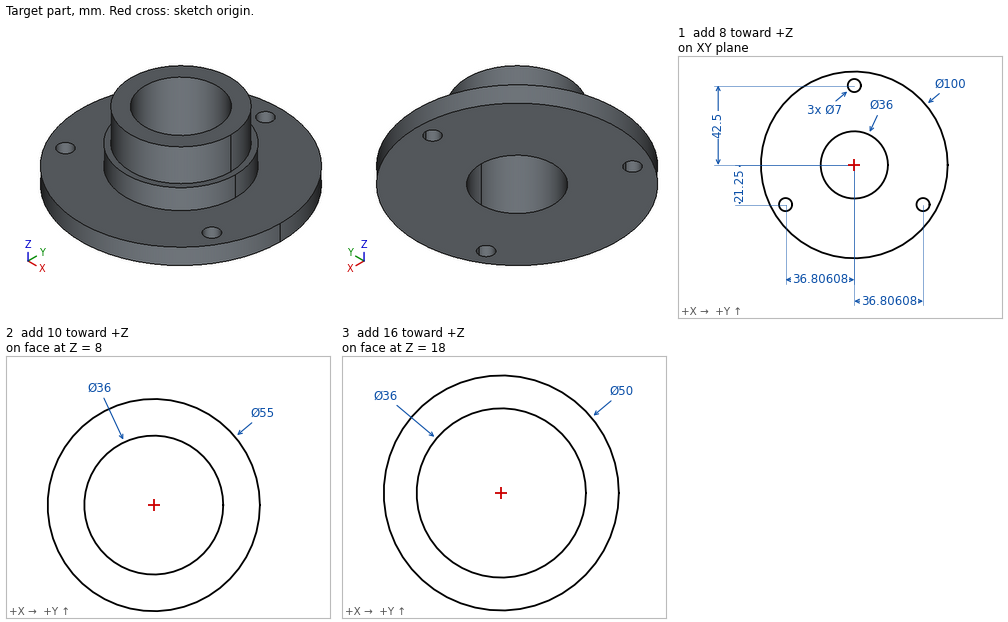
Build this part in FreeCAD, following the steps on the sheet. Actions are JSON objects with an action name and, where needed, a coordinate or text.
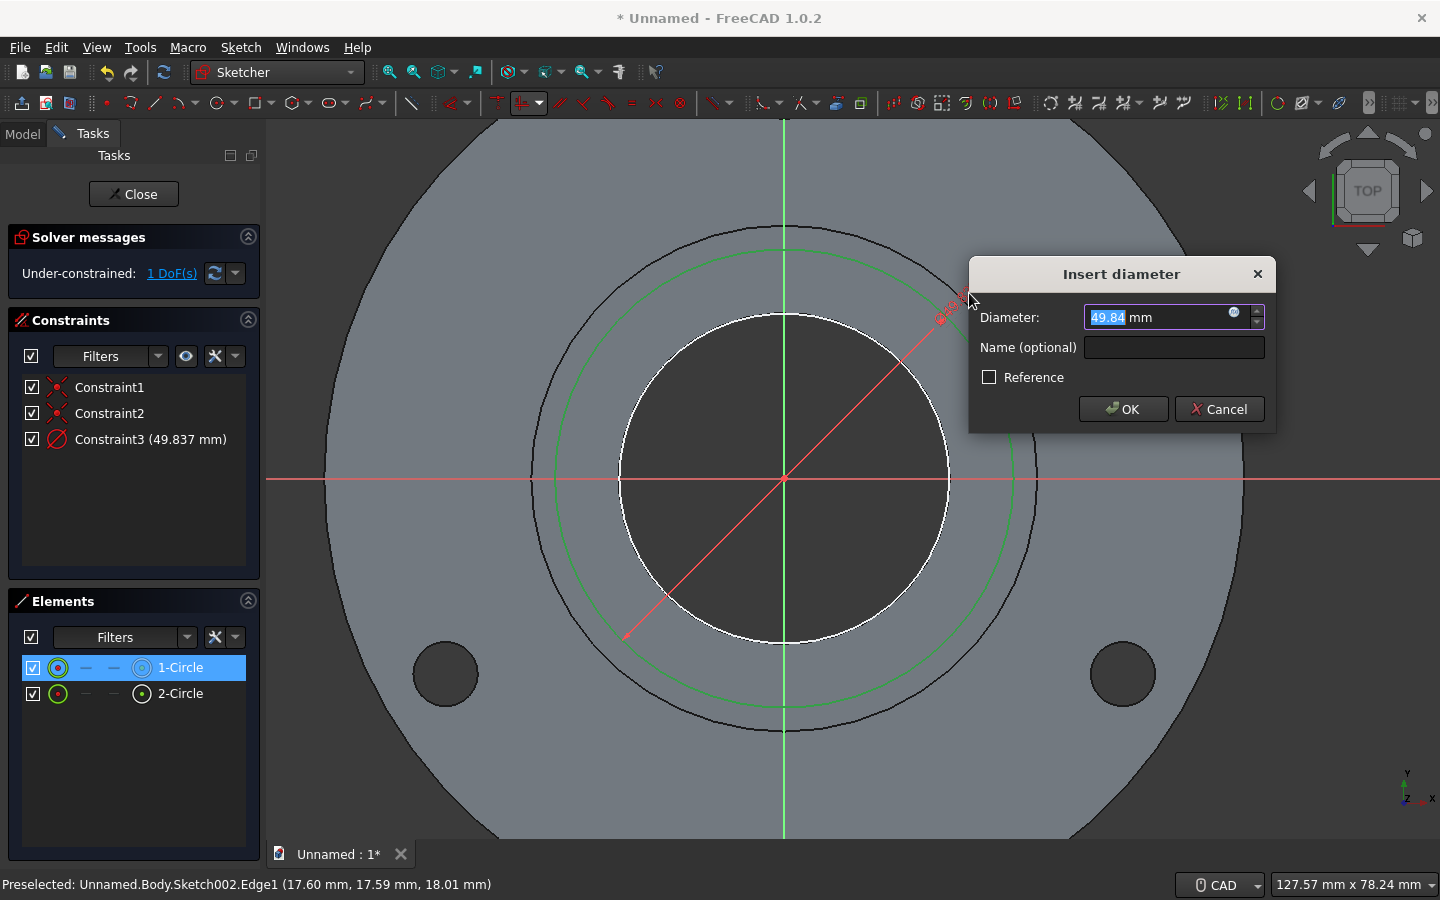
{"action": "type", "text": "50"}
{"action": "key", "text": "Return"}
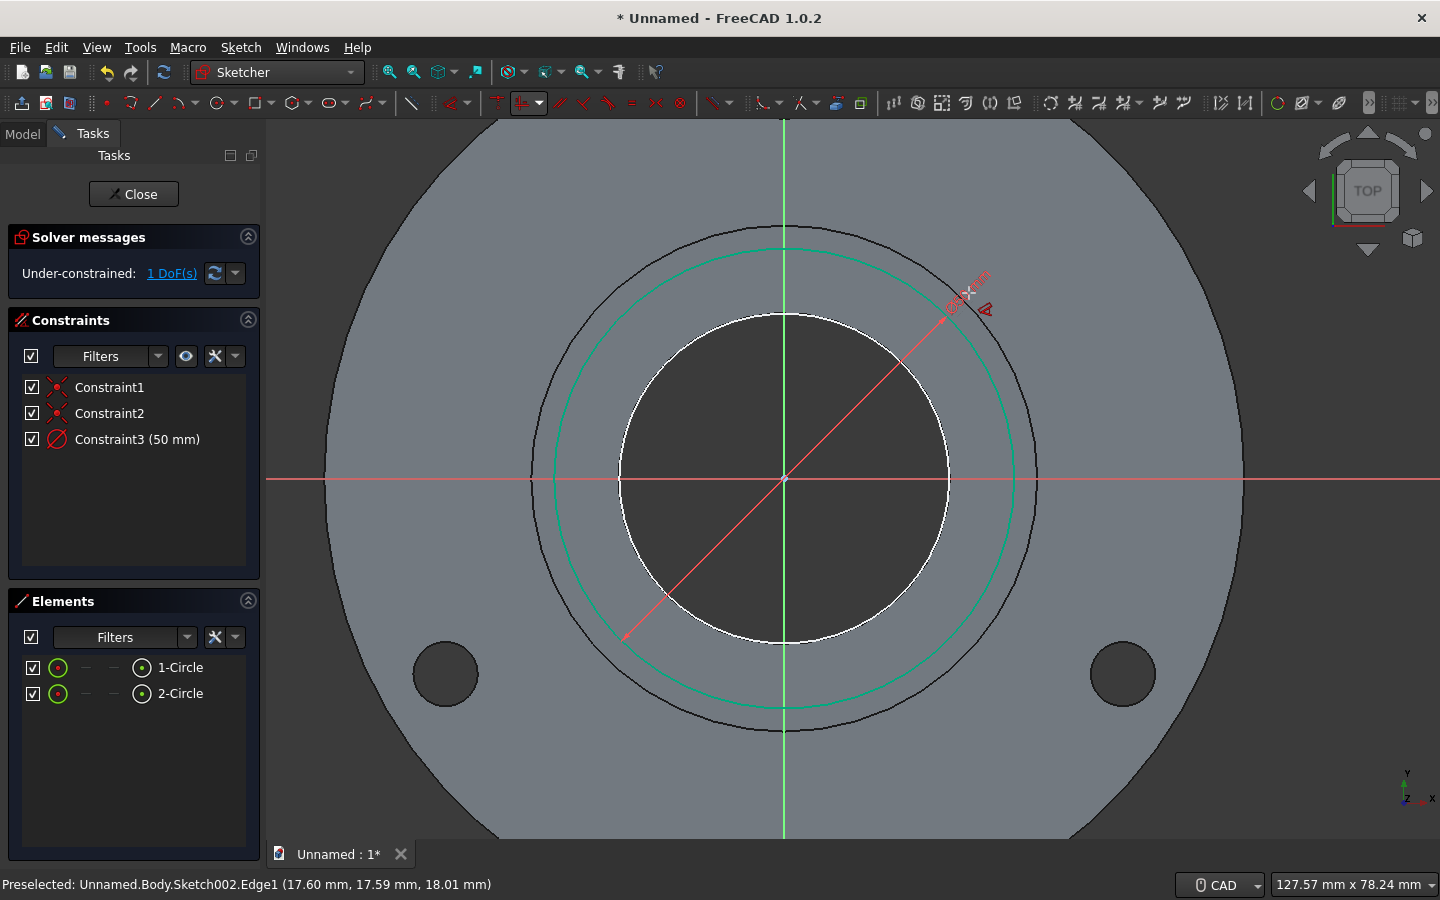
{"action": "left_click", "coordinate": [901, 362]}
{"action": "left_click", "coordinate": [924, 339]}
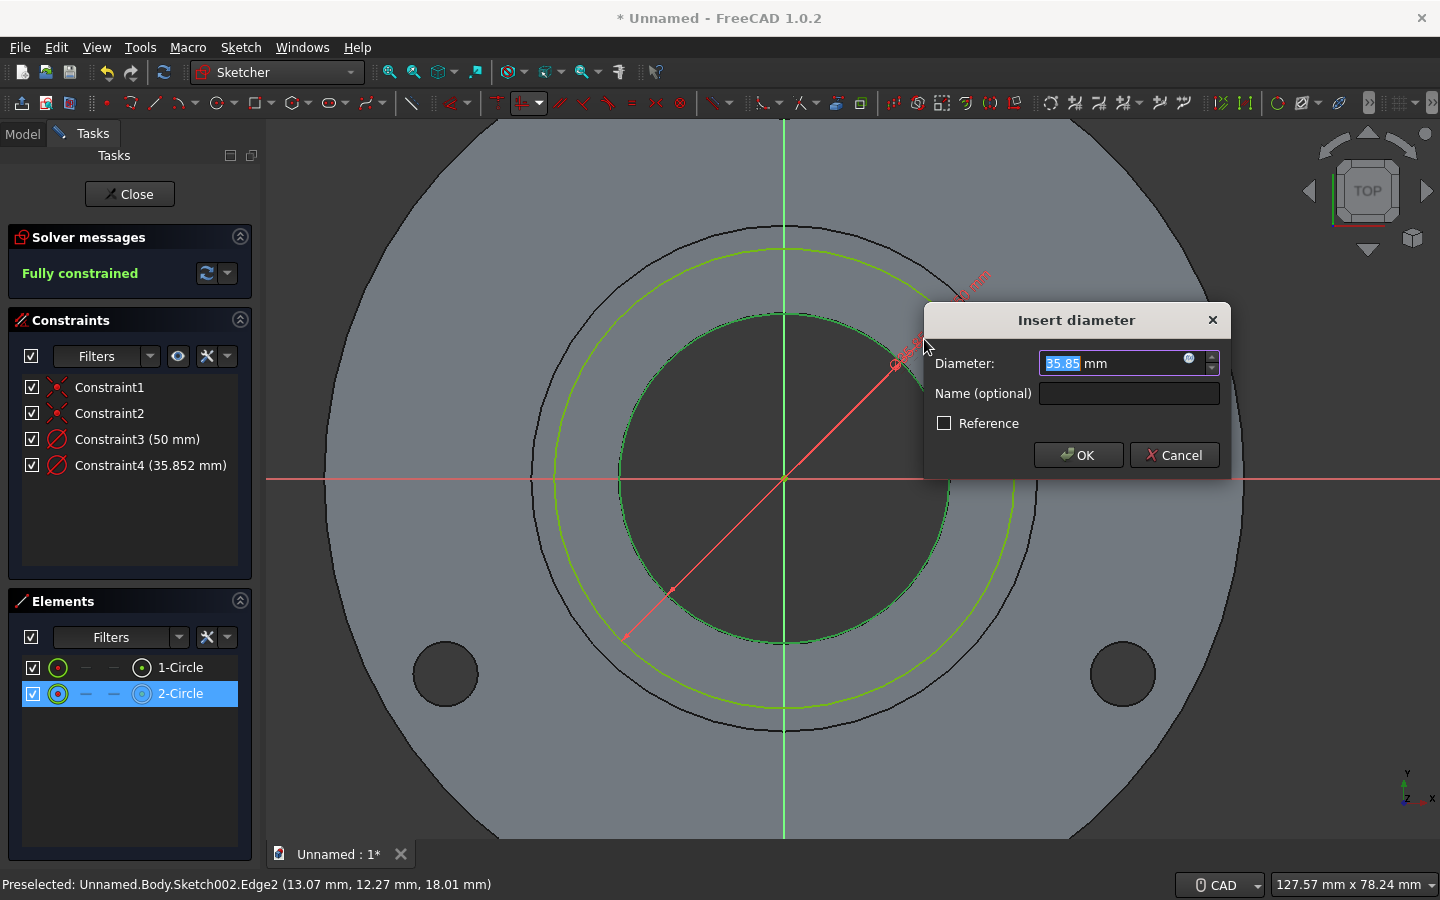
{"action": "type", "text": "36"}
{"action": "key", "text": "Return"}
{"action": "key", "text": "Escape"}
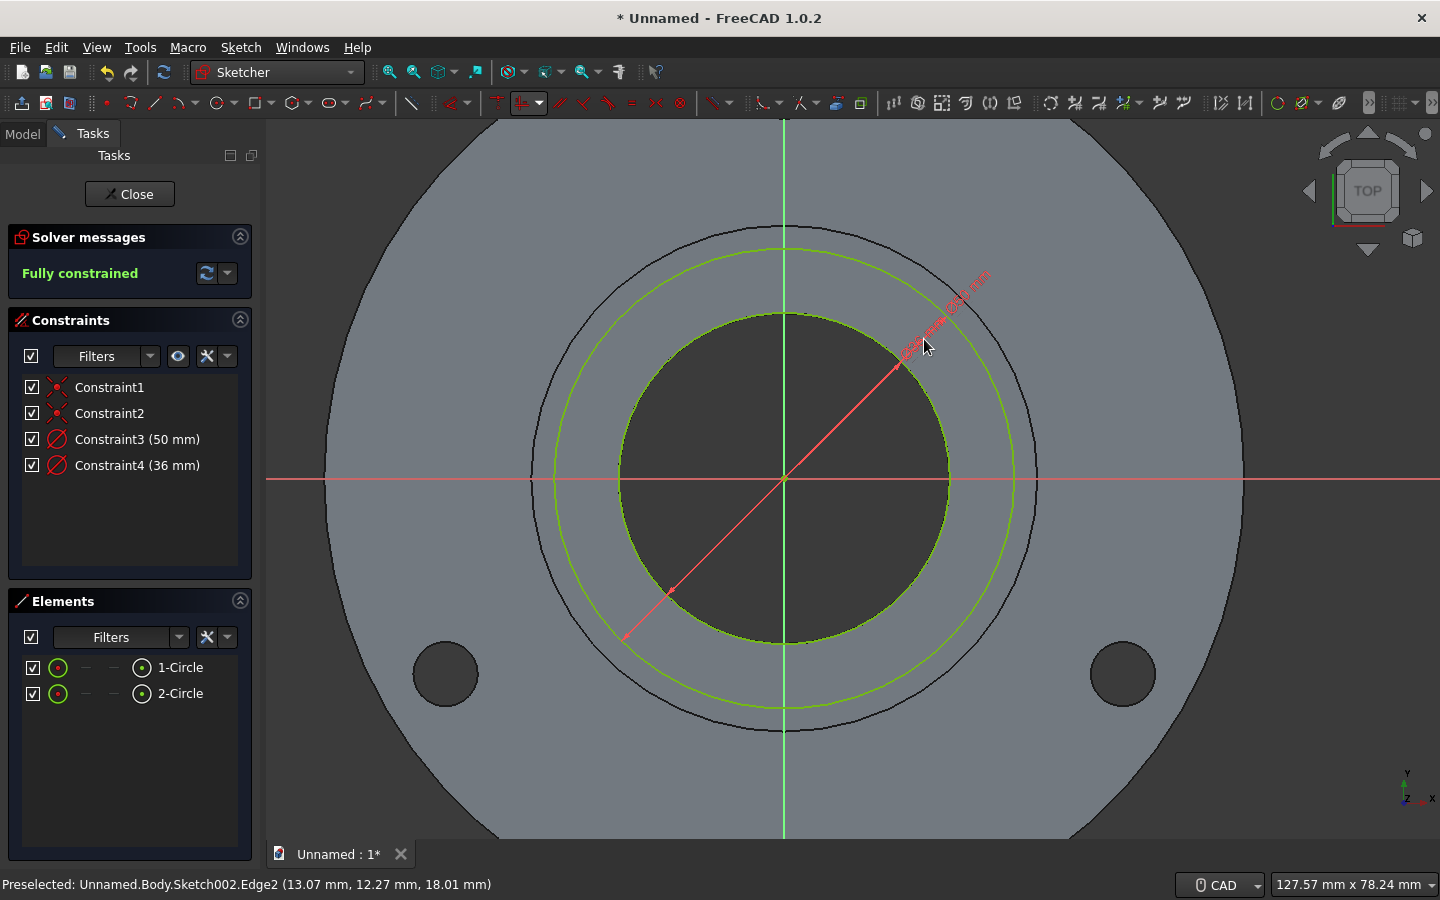
{"action": "left_click", "coordinate": [130, 194]}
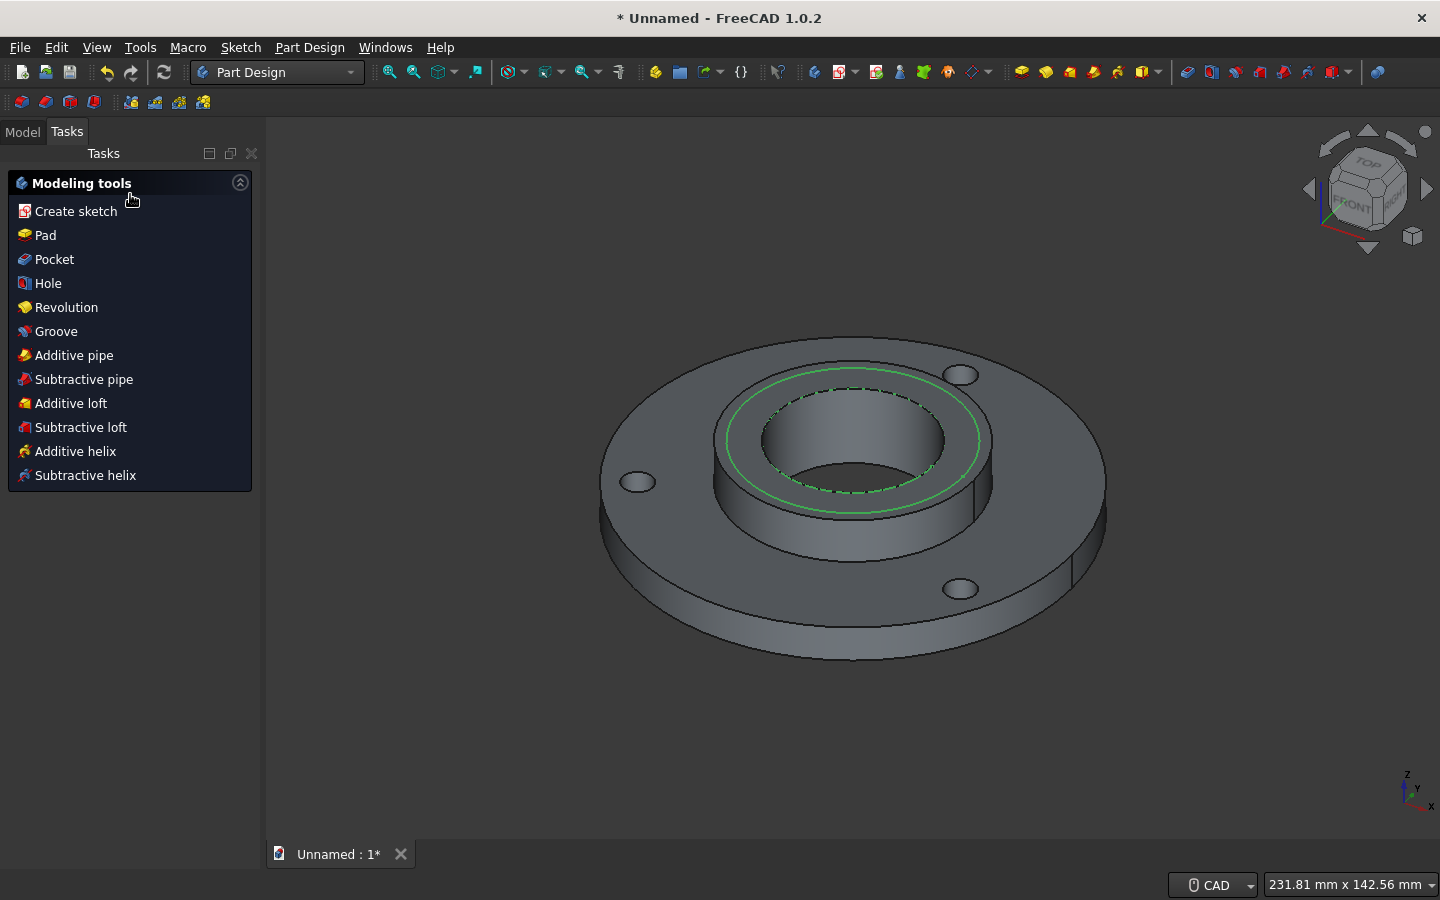
{"action": "left_click", "coordinate": [1022, 72]}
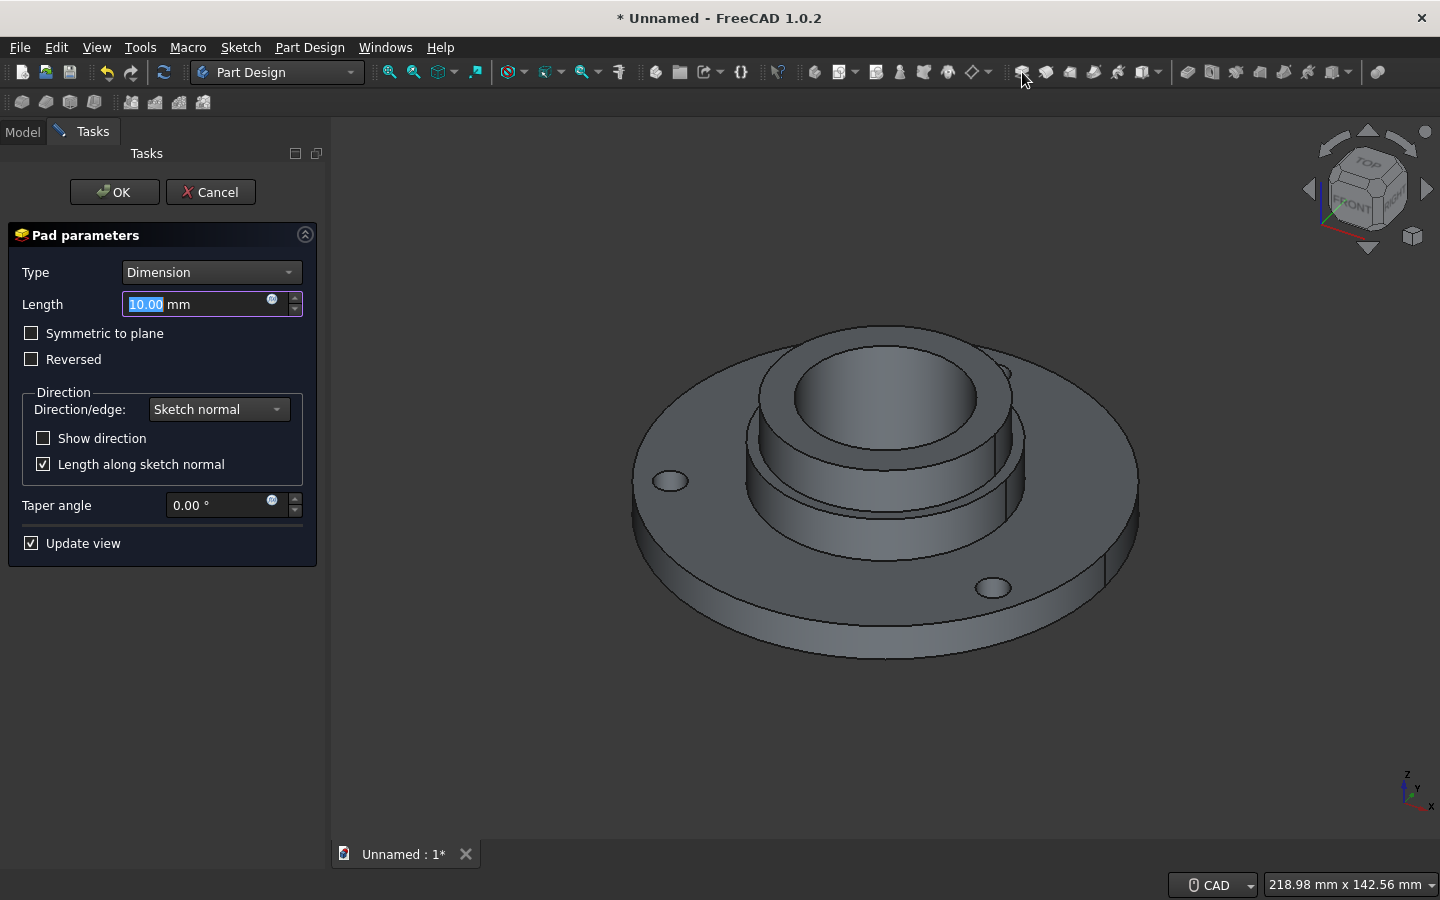
{"action": "type", "text": "16"}
{"action": "key", "text": "Tab"}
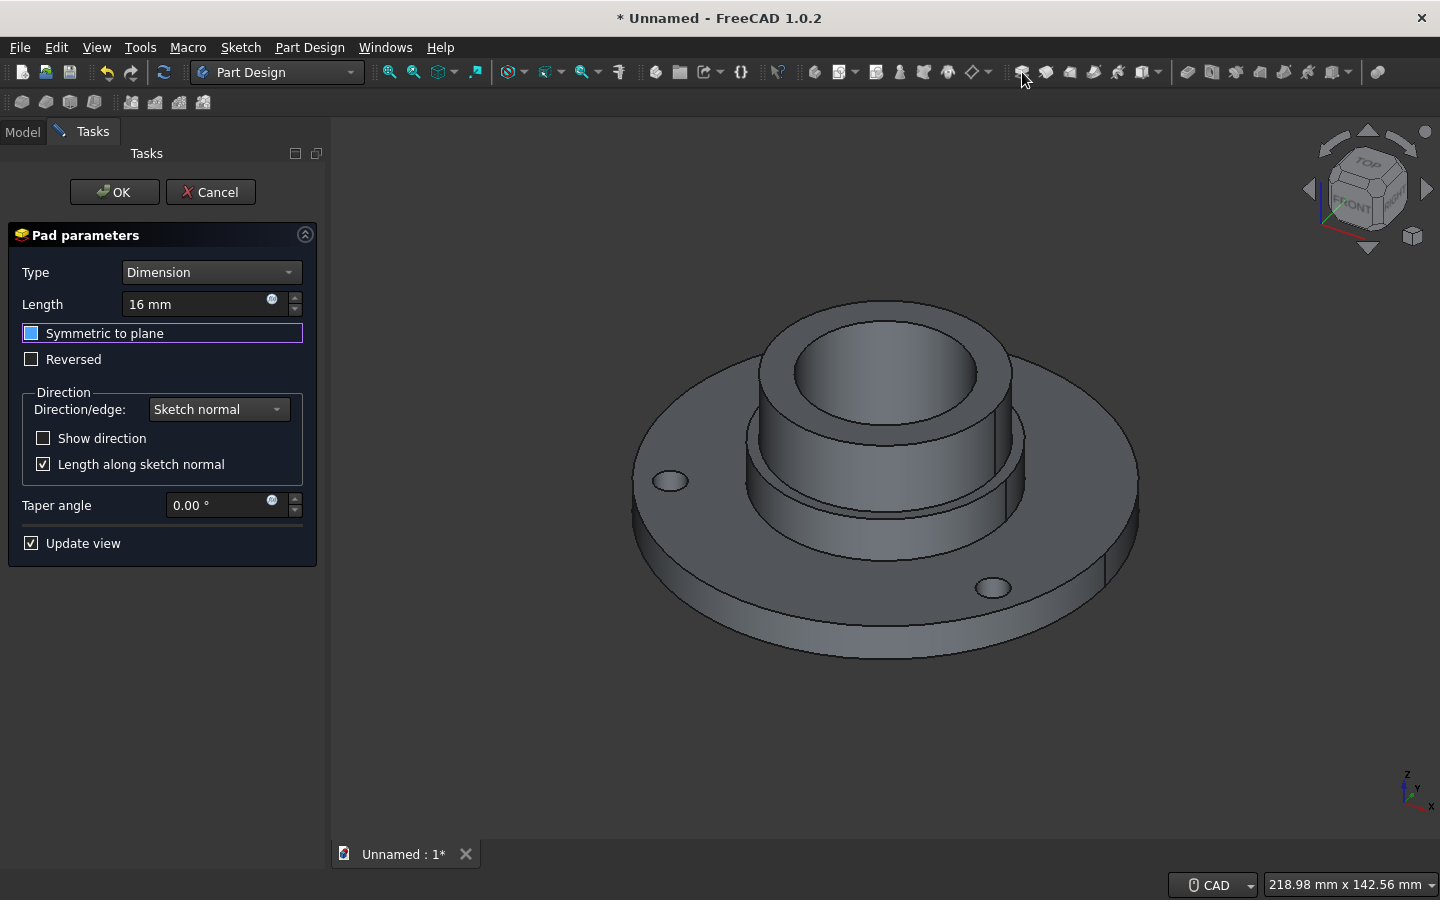
{"action": "left_click", "coordinate": [115, 192]}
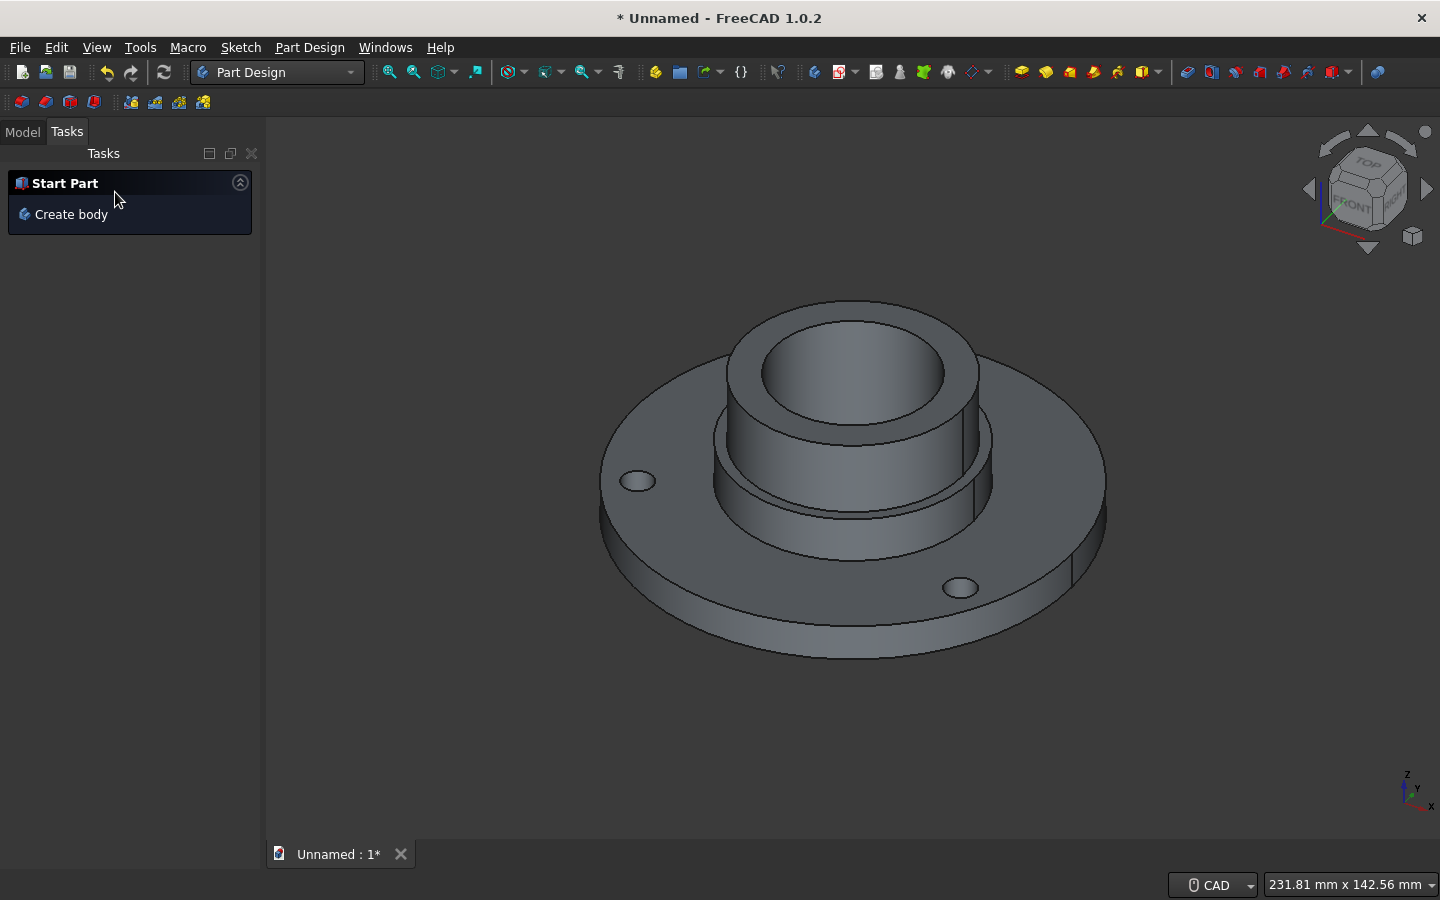
{"action": "key", "text": "0"}